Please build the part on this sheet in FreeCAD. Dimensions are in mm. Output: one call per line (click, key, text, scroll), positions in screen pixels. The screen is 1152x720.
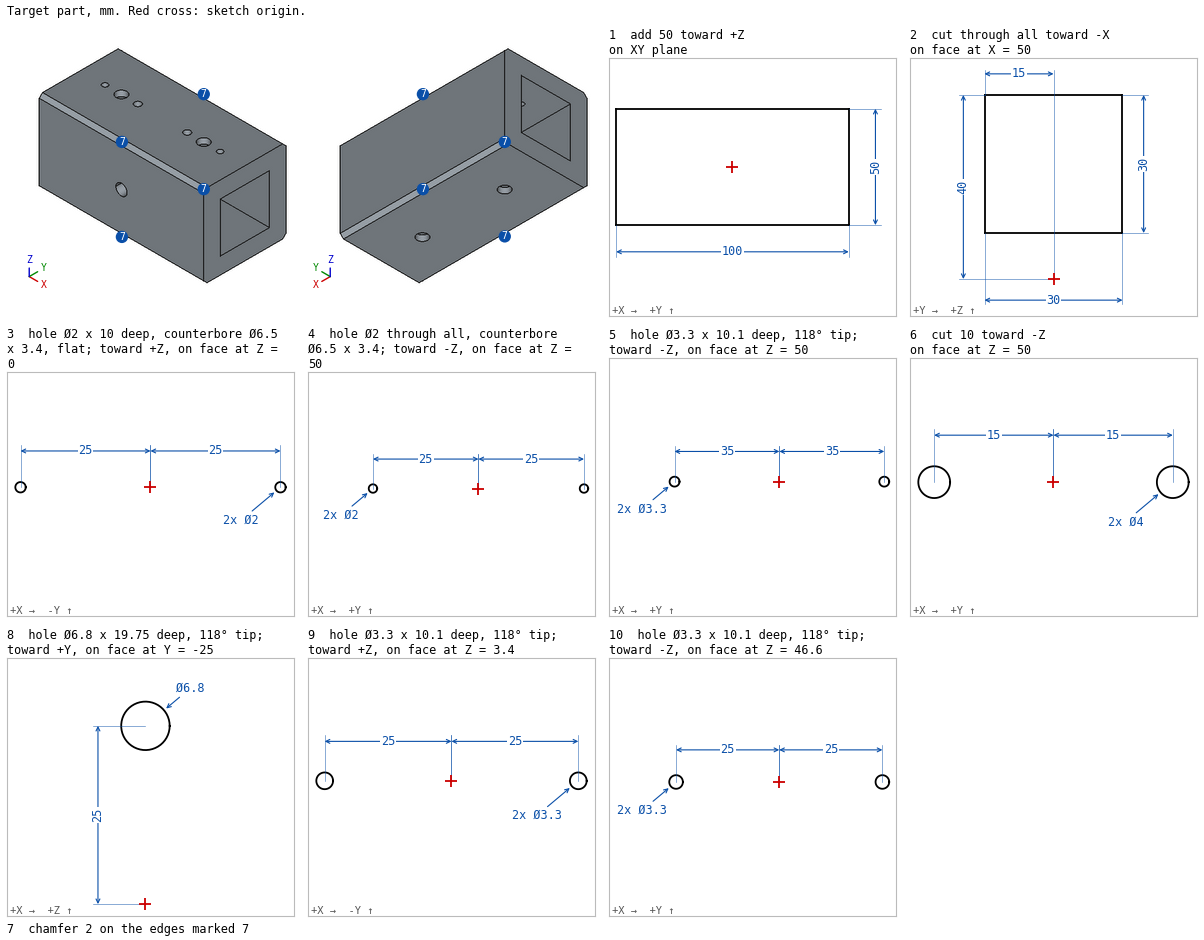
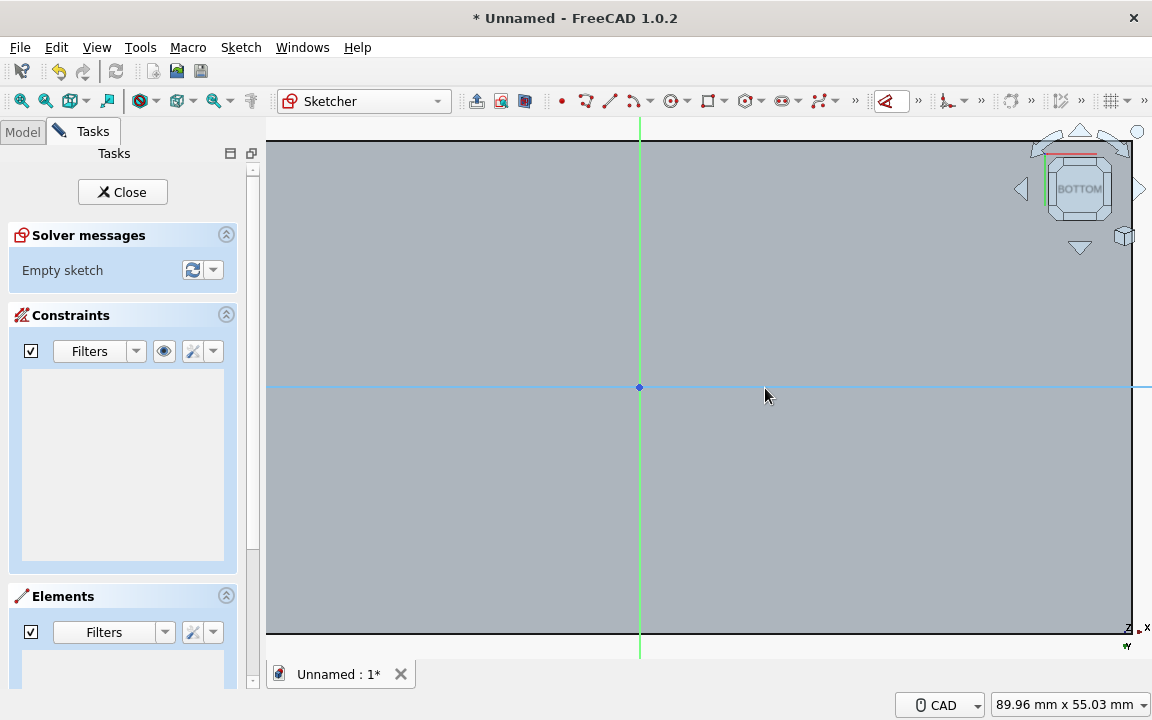
click(672, 102)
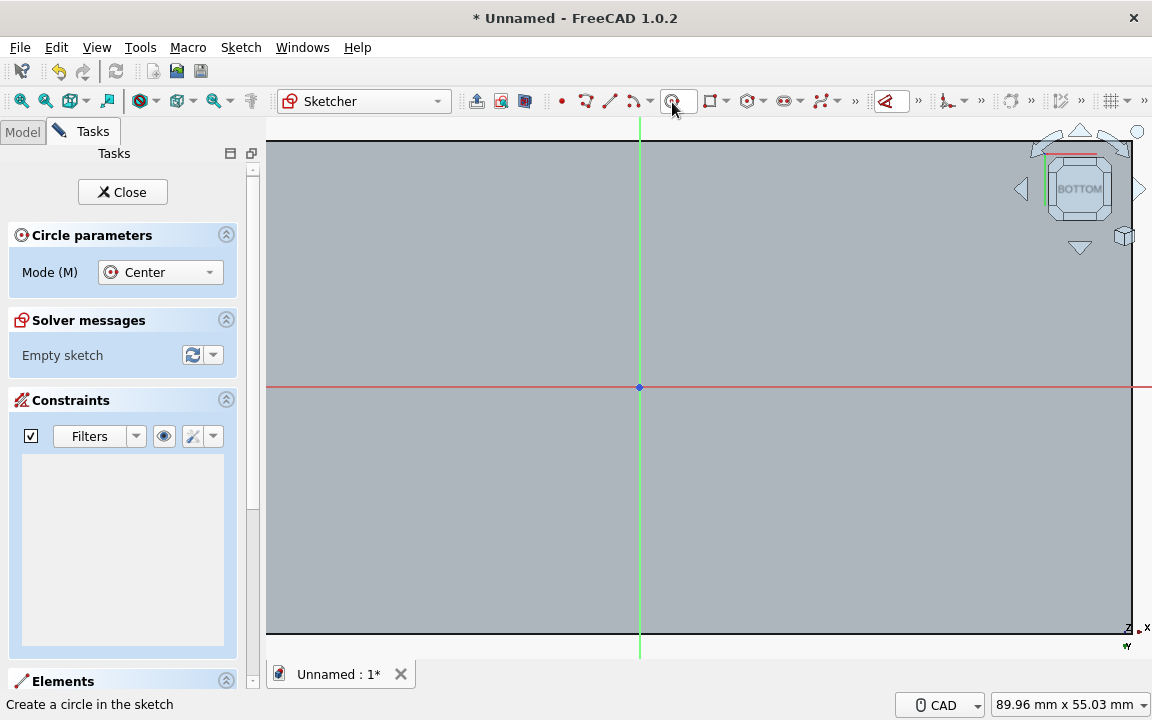
scroll(886, 387, up, 5)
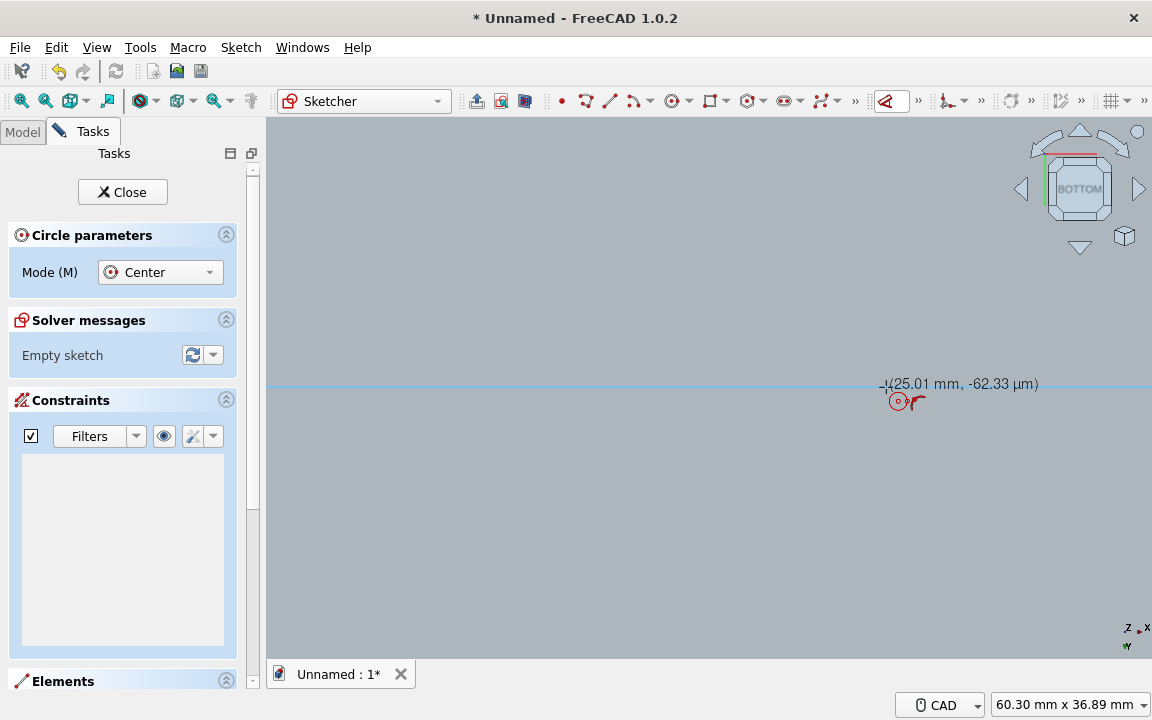
click(885, 387)
move(903, 368)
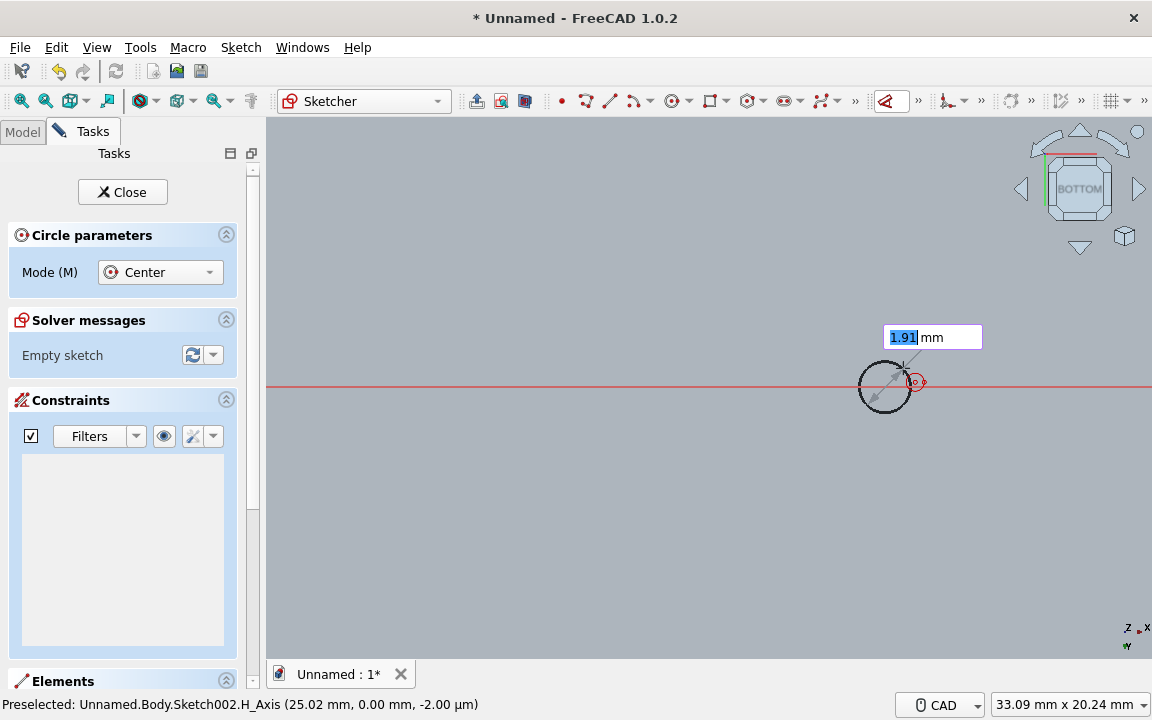
text(2)
key(Return)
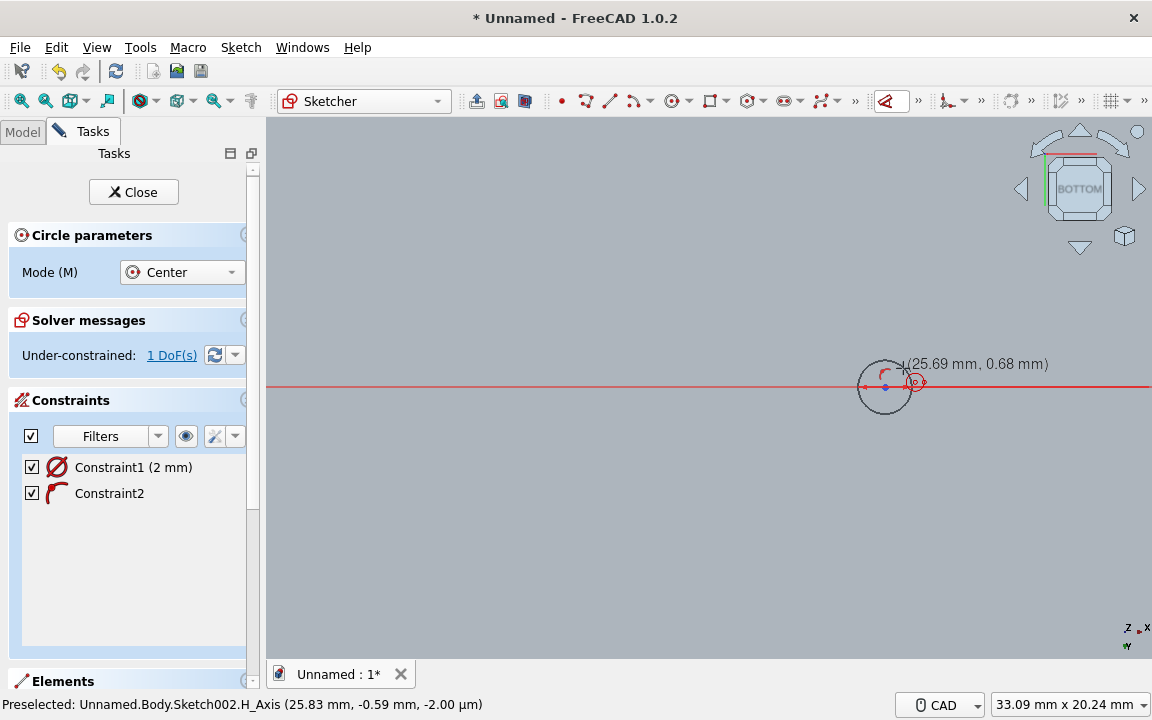
scroll(888, 388, down, 5)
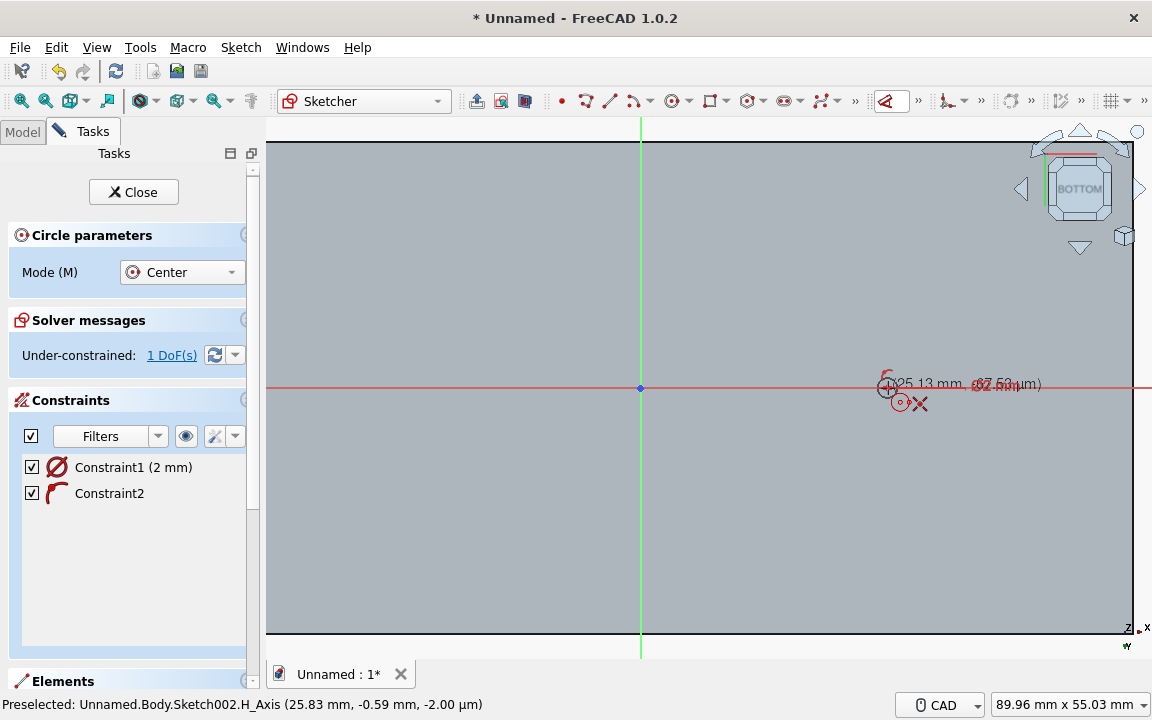
scroll(395, 388, up, 5)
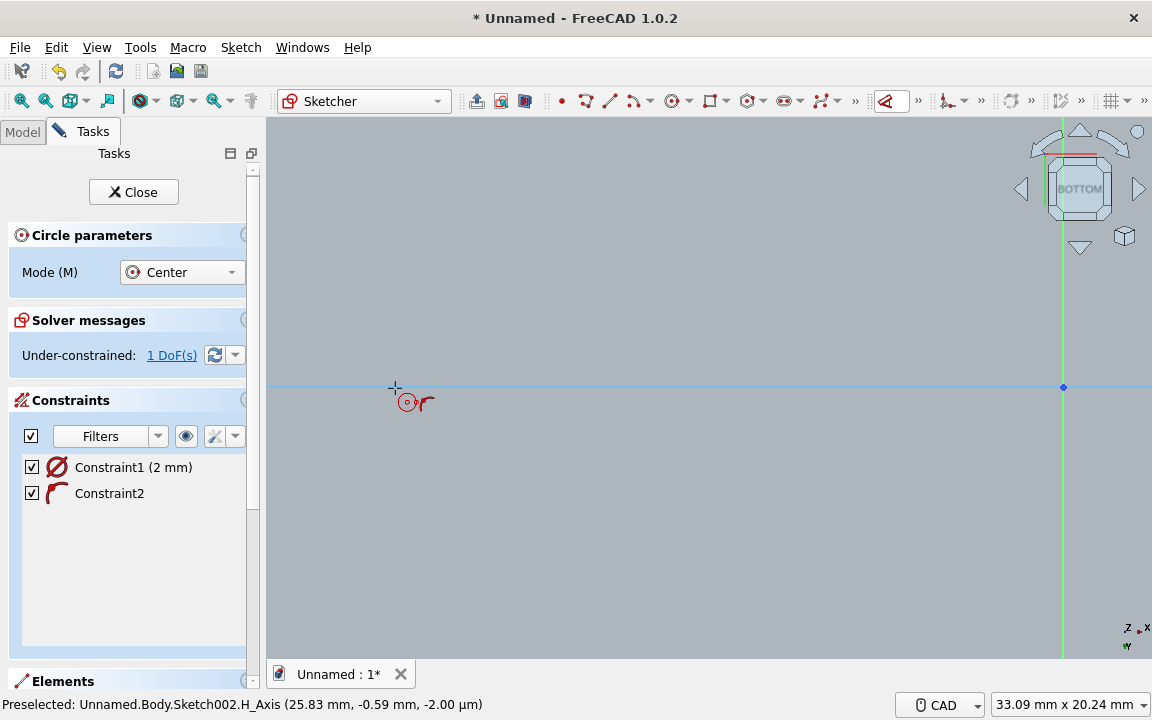
click(394, 387)
move(413, 368)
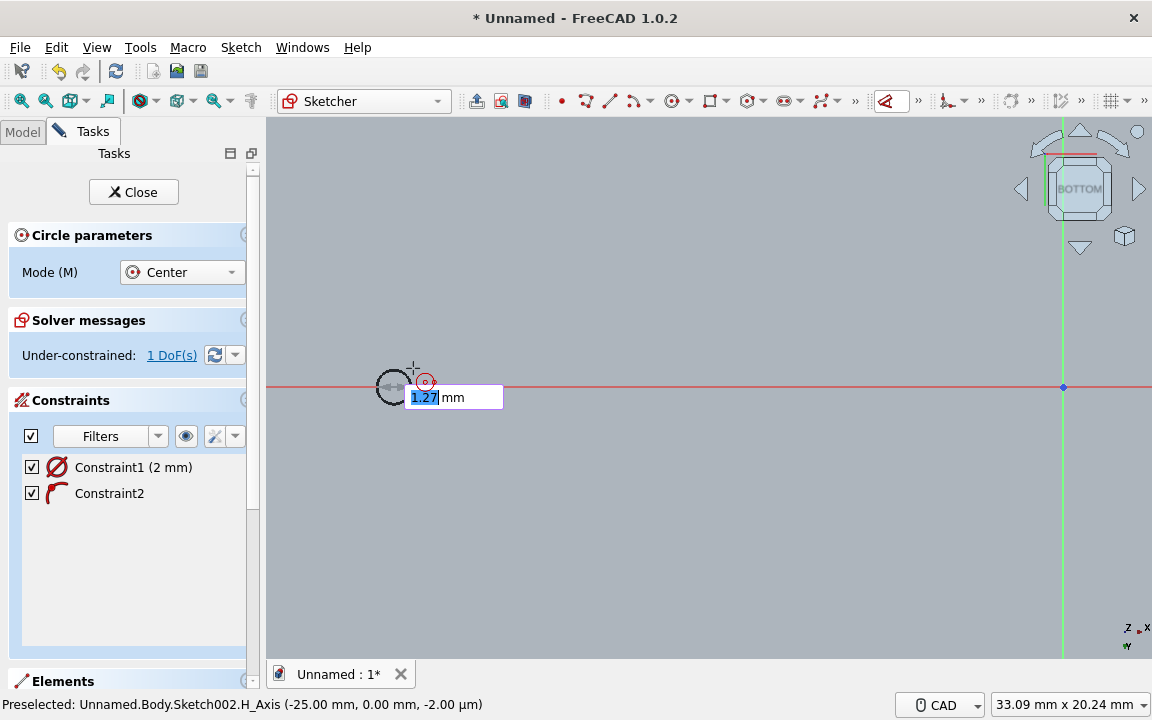
text(2)
key(Return)
key(Escape)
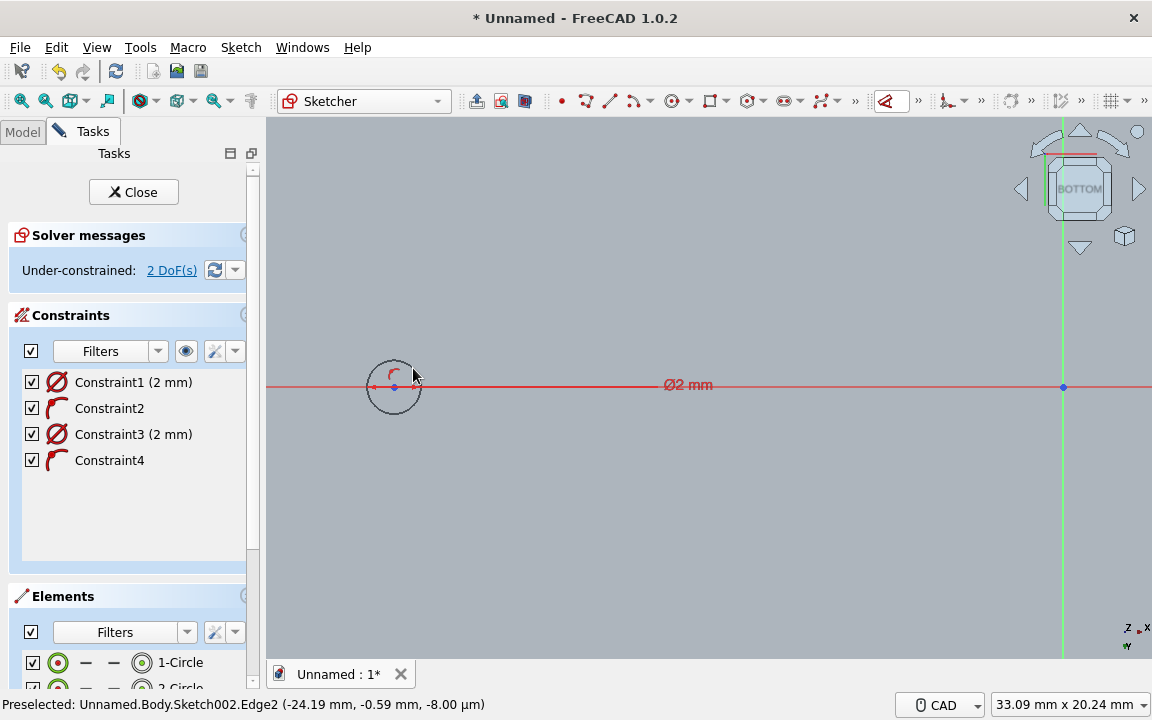
scroll(394, 388, down, 5)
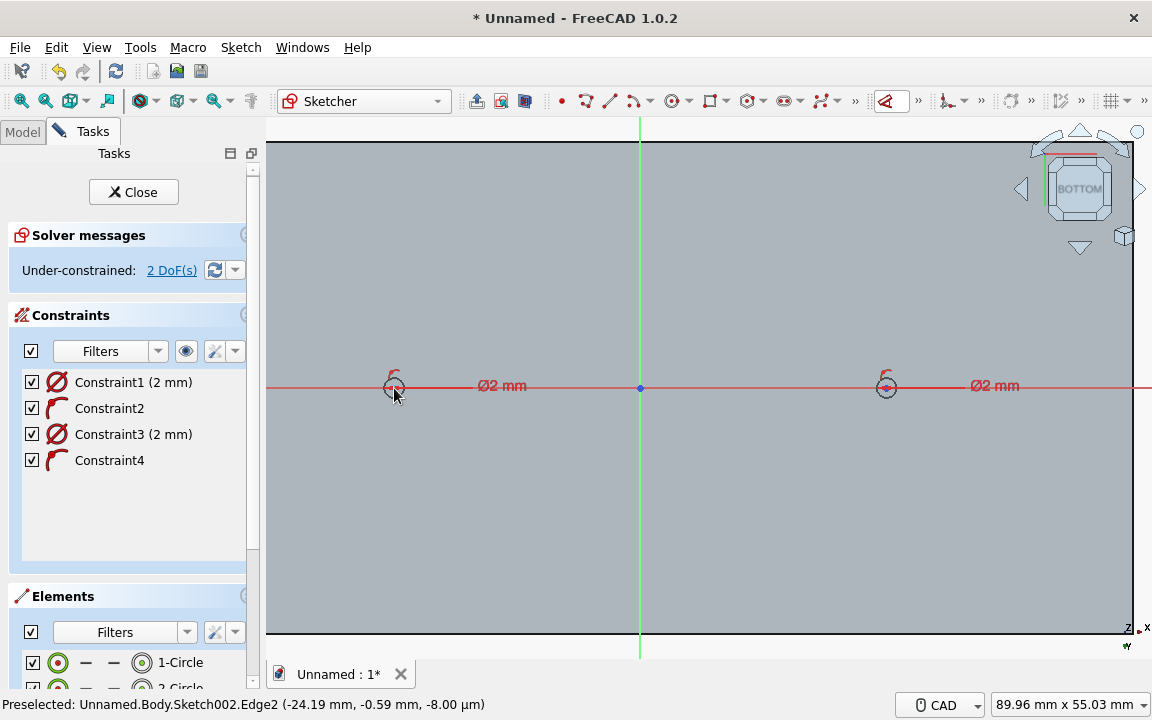
click(887, 388)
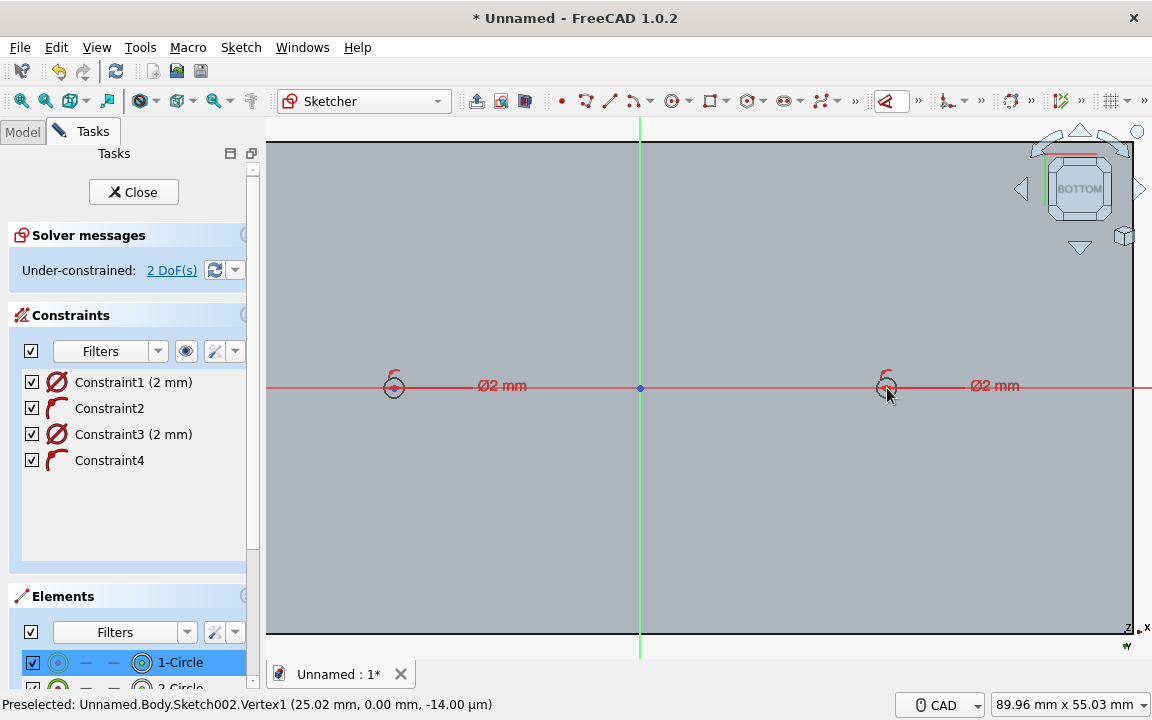
click(904, 102)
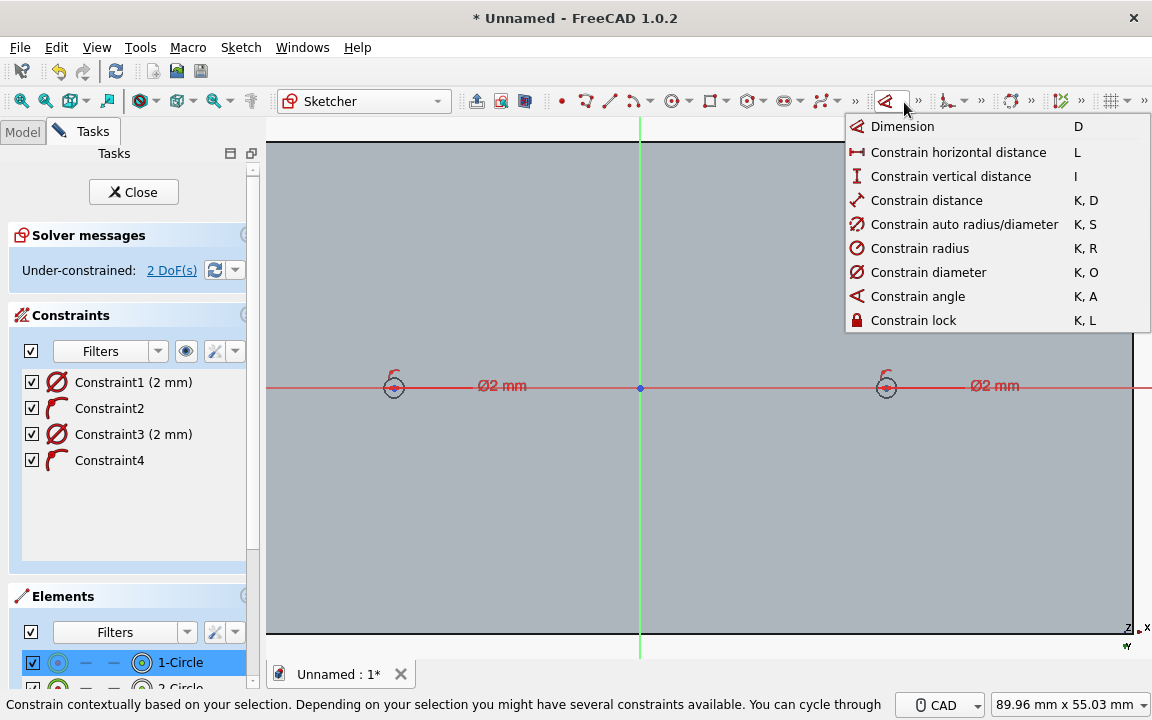
click(998, 152)